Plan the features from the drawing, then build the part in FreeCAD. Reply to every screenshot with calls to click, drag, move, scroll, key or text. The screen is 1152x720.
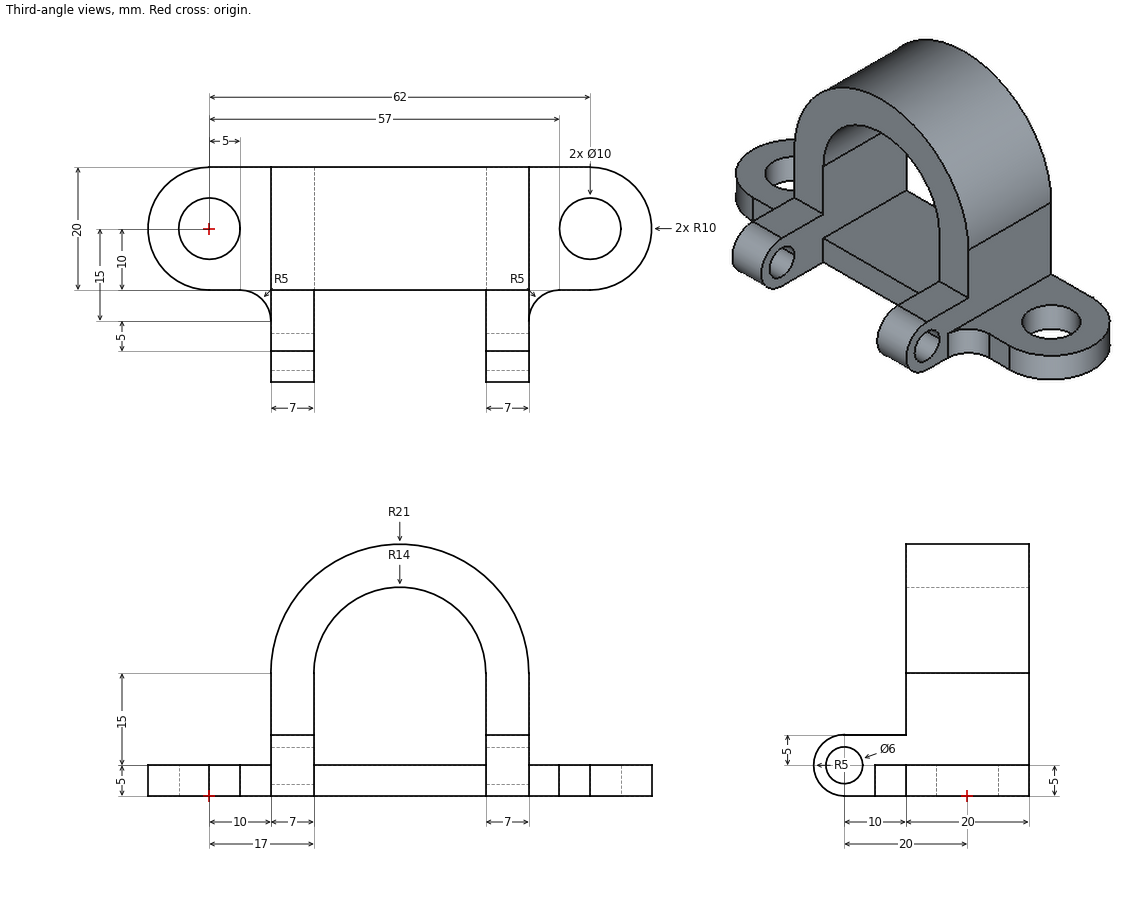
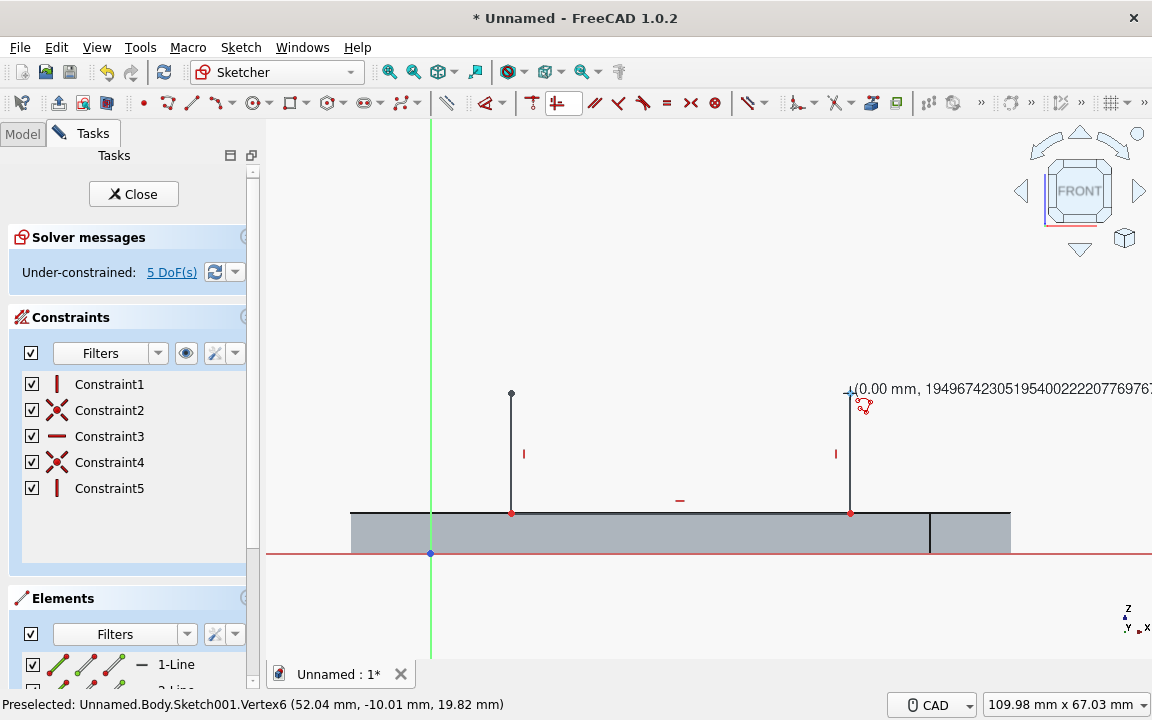
click(216, 104)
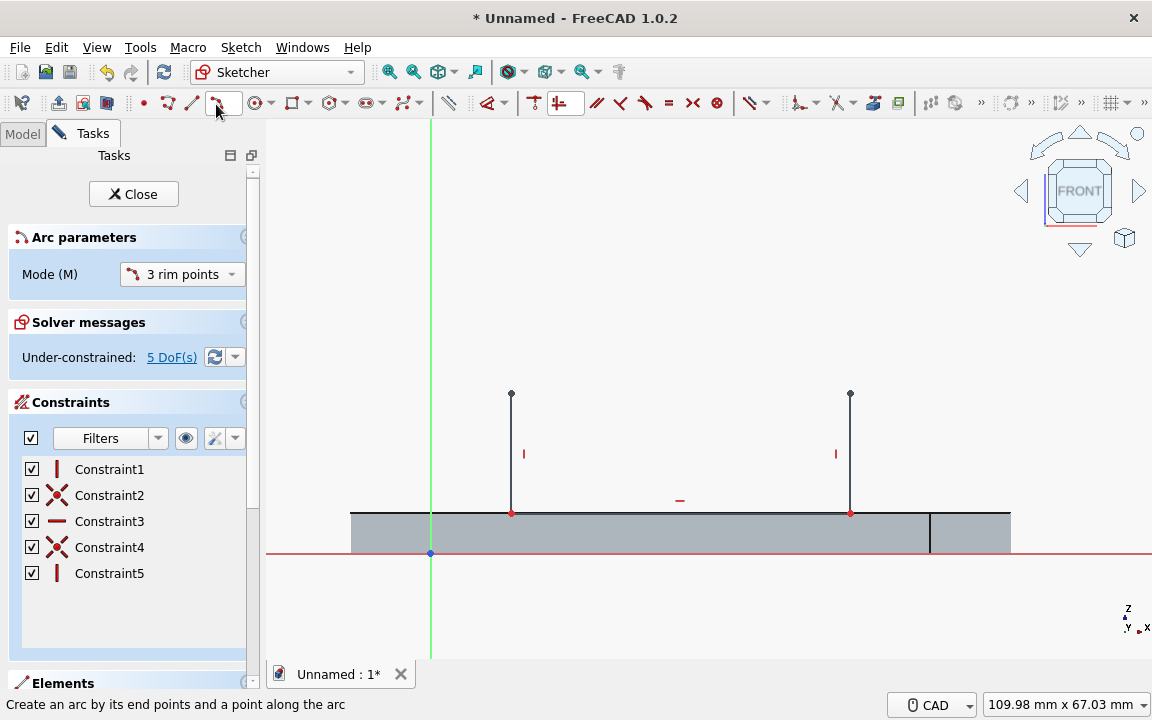
click(850, 394)
click(511, 394)
click(681, 223)
key(Escape)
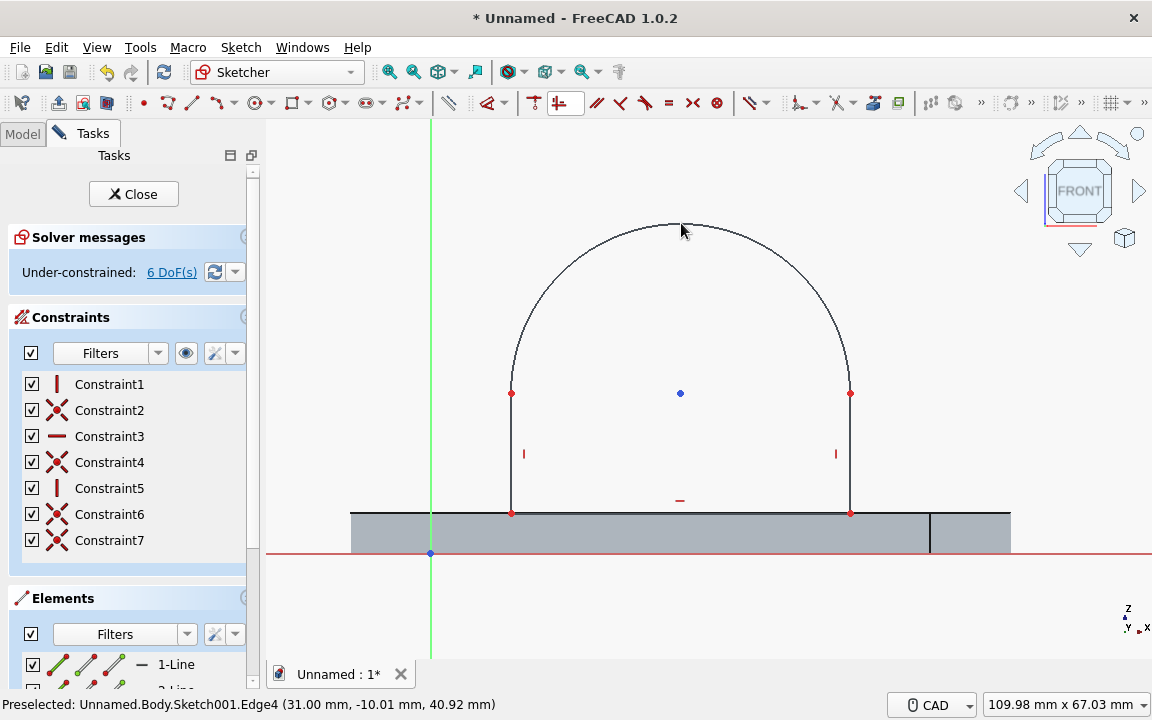
click(511, 430)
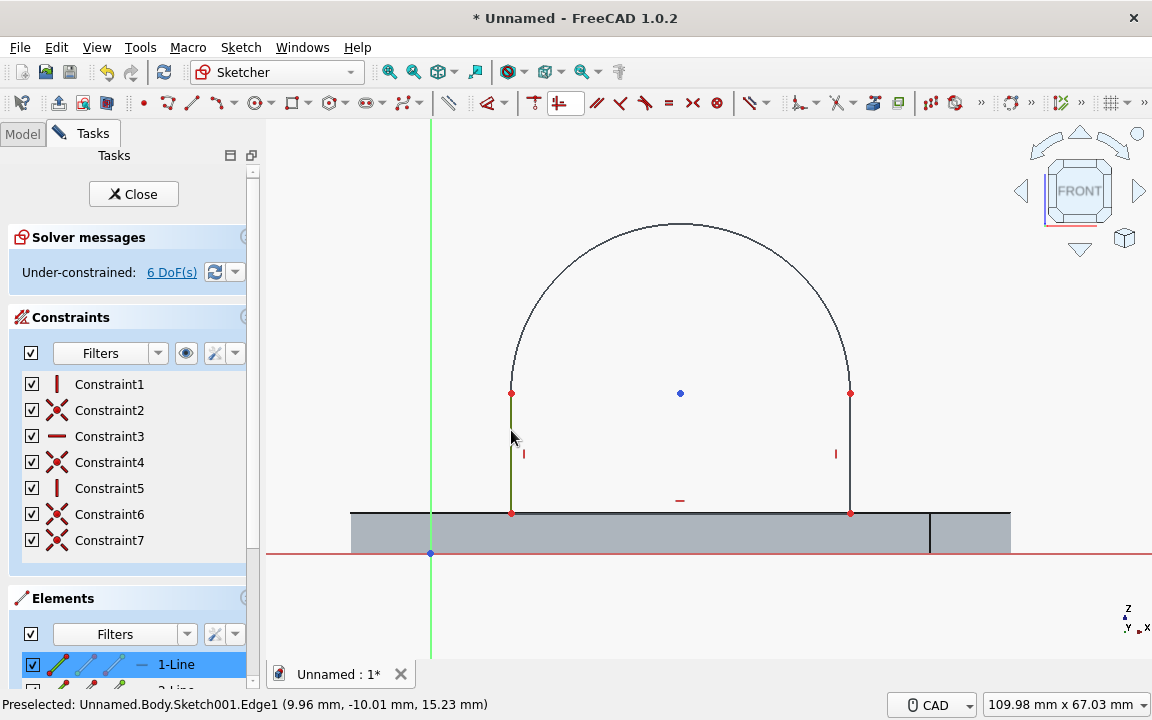
click(780, 256)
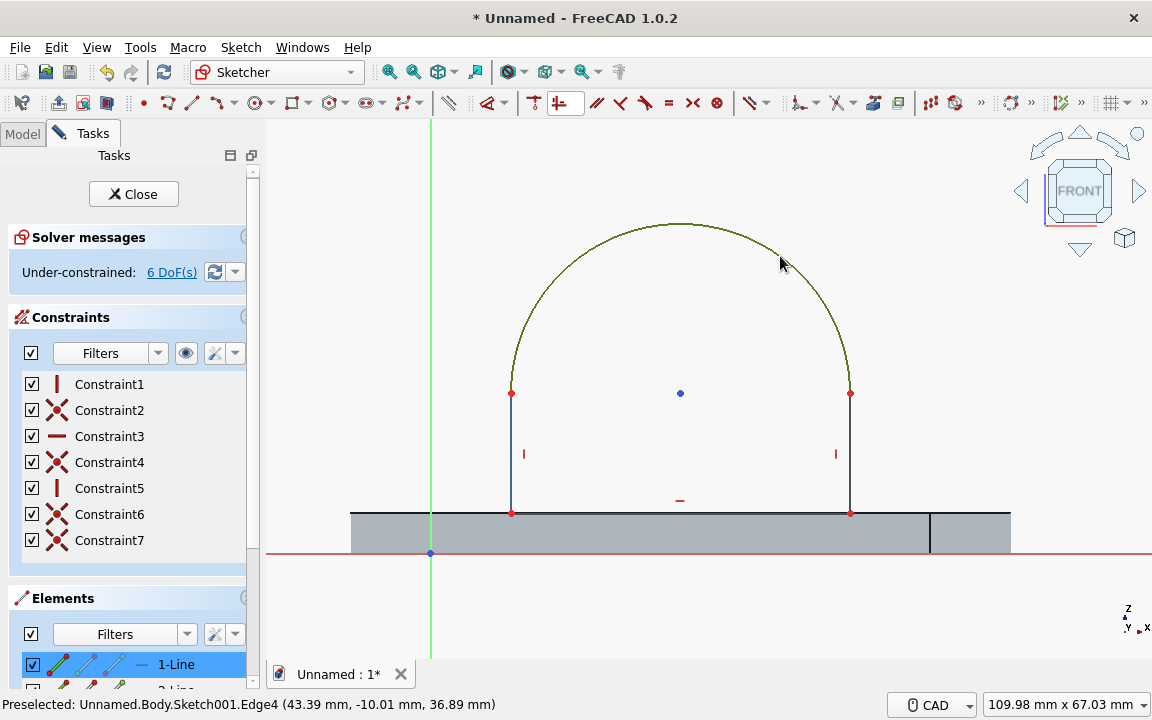
click(646, 104)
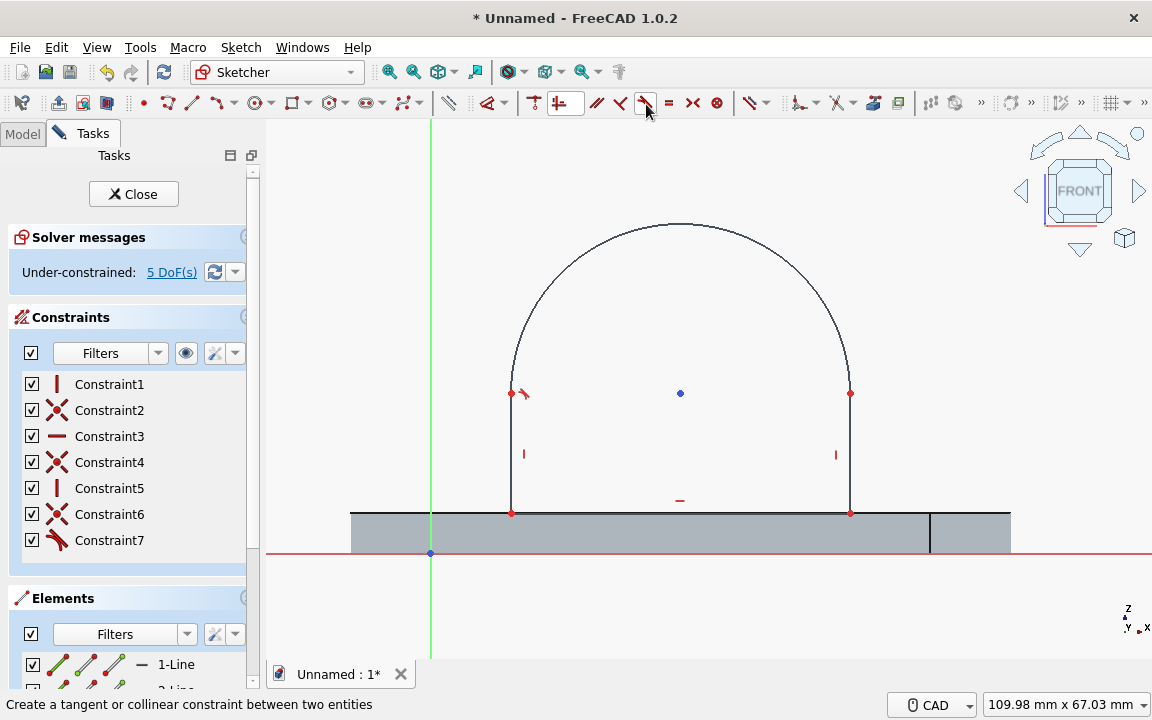
click(850, 478)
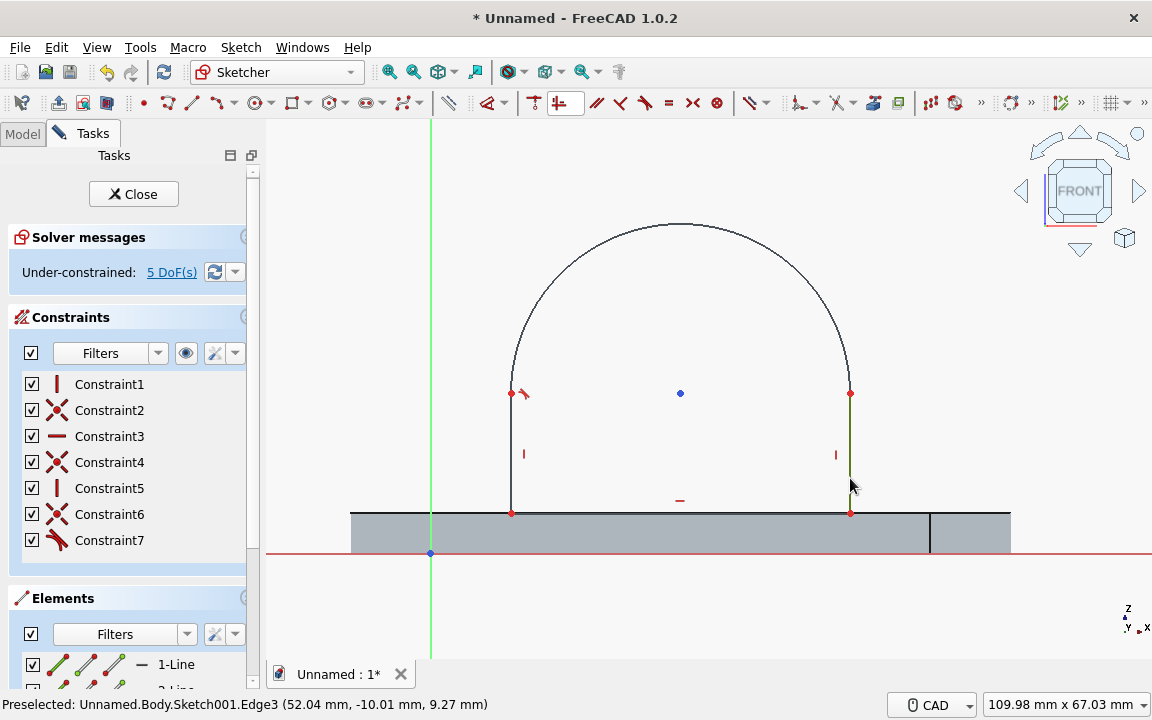
click(780, 257)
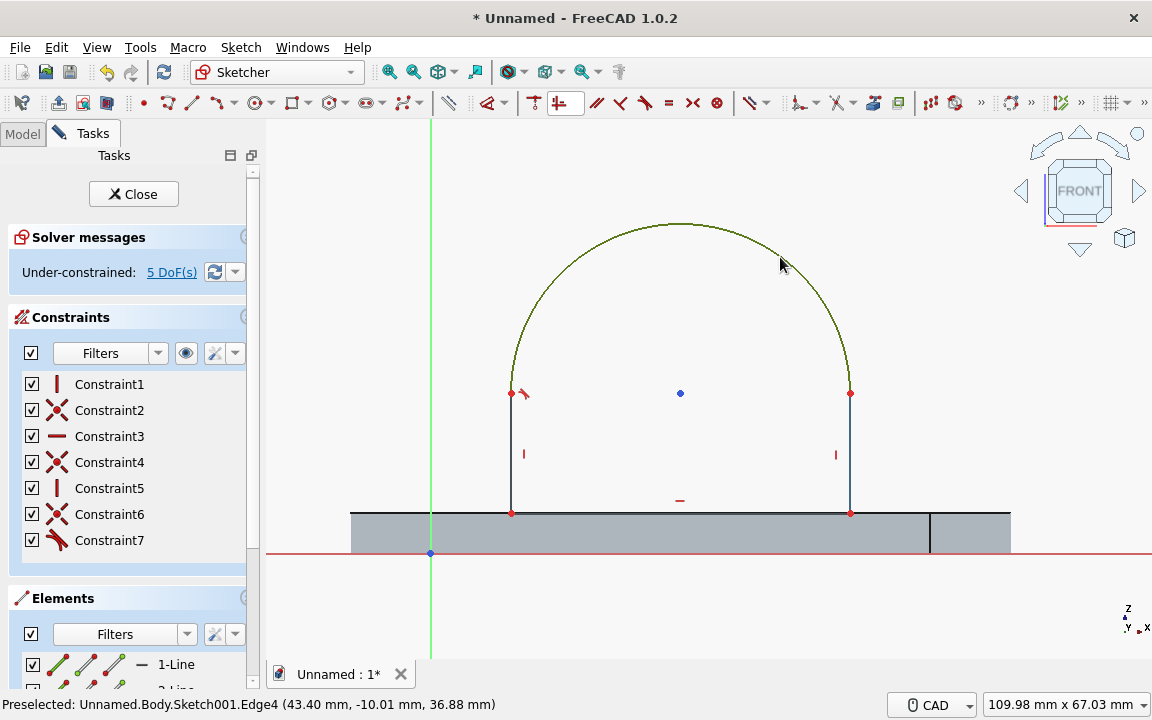
click(646, 104)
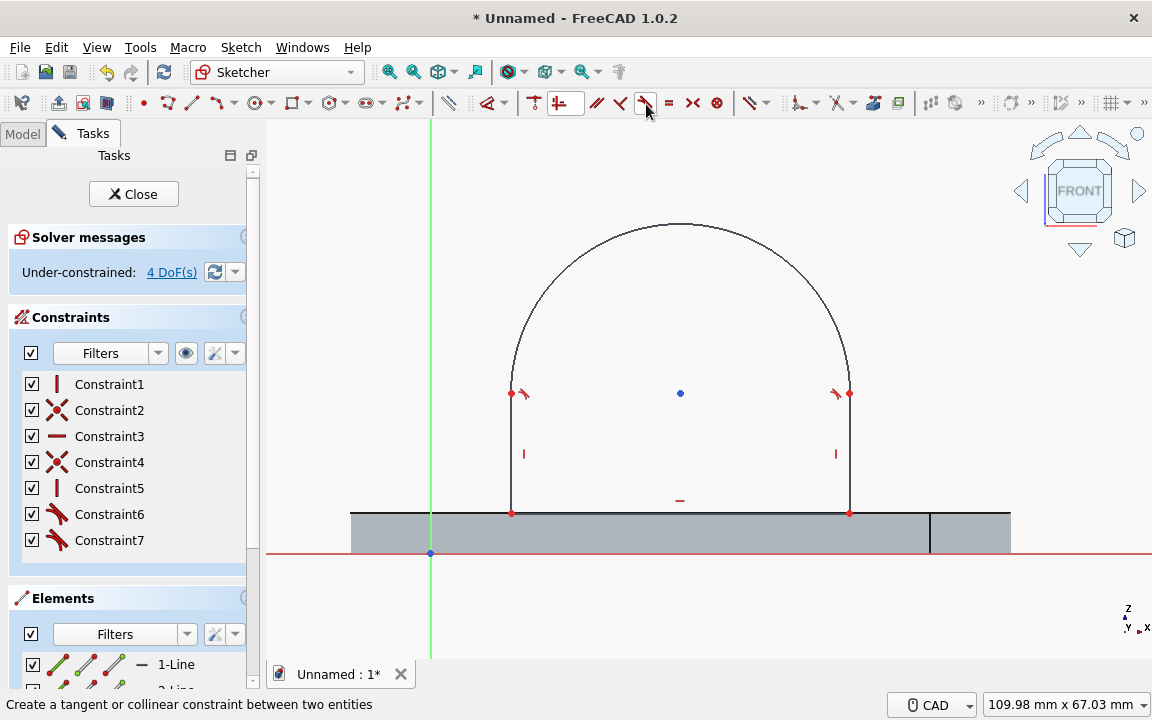
key(d)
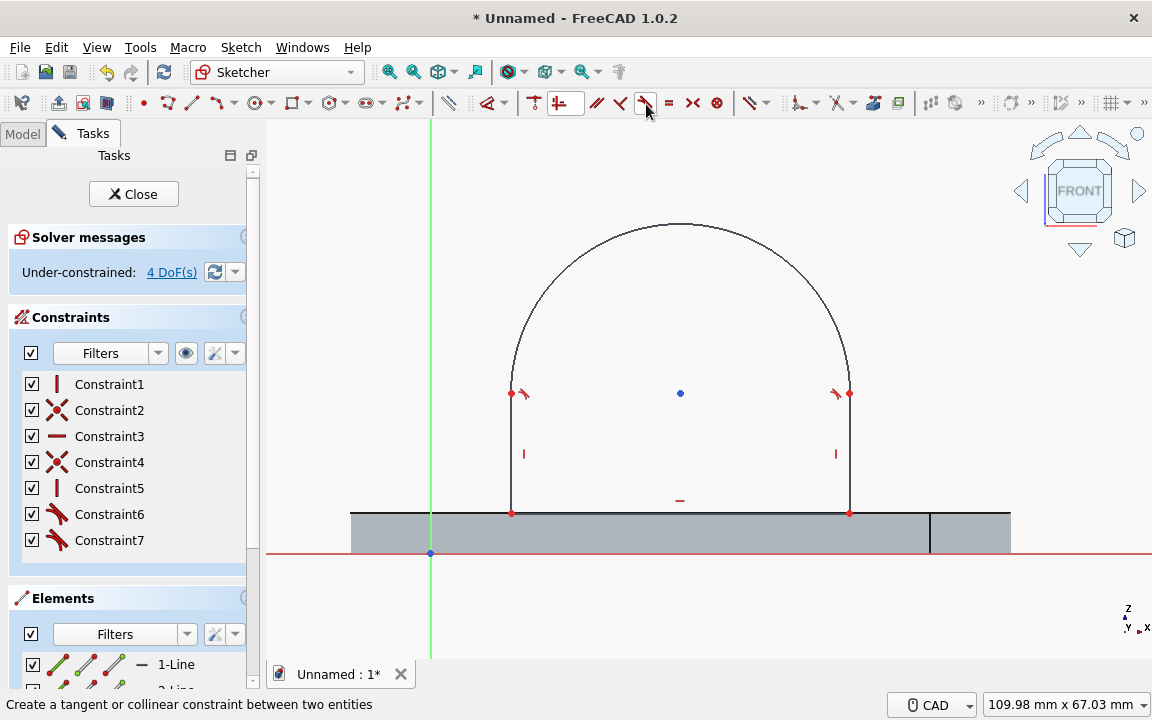
click(780, 256)
click(799, 230)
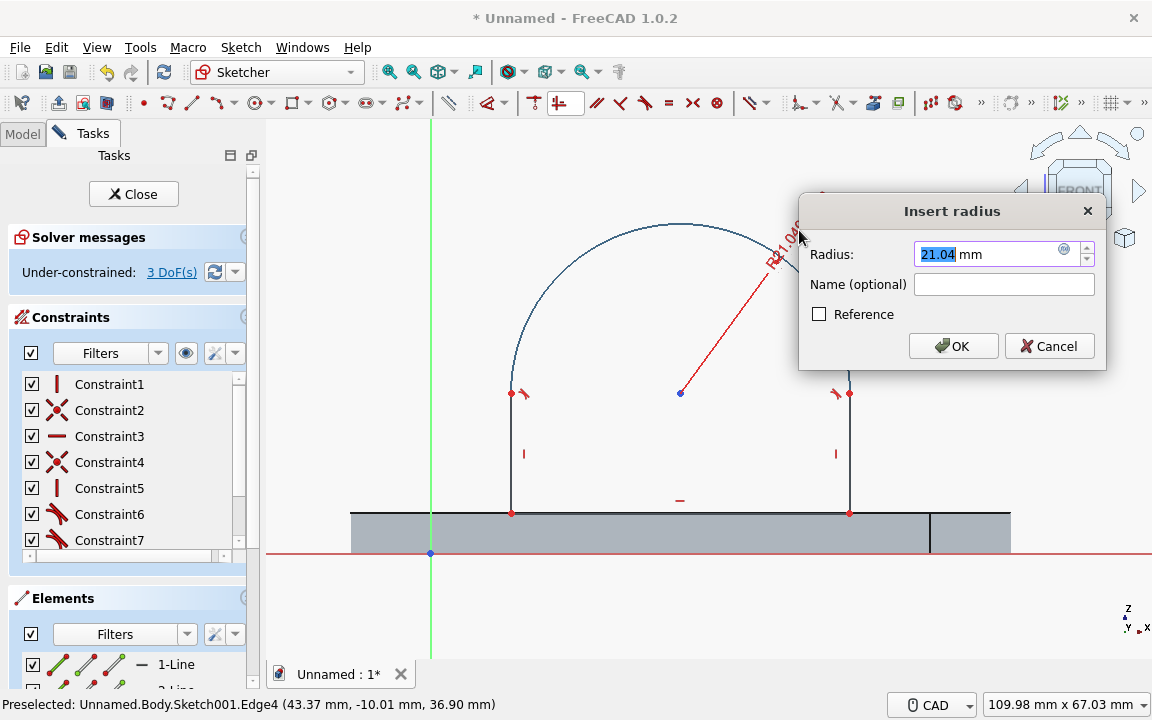
text(21)
key(Return)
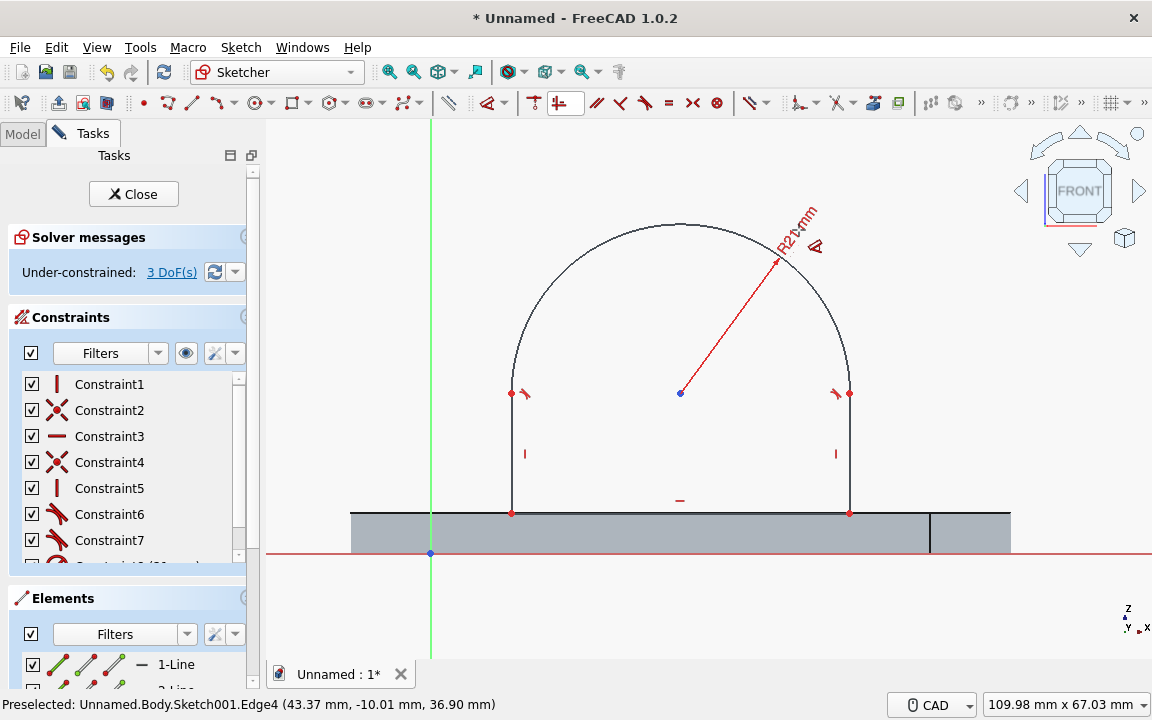
click(512, 430)
click(478, 454)